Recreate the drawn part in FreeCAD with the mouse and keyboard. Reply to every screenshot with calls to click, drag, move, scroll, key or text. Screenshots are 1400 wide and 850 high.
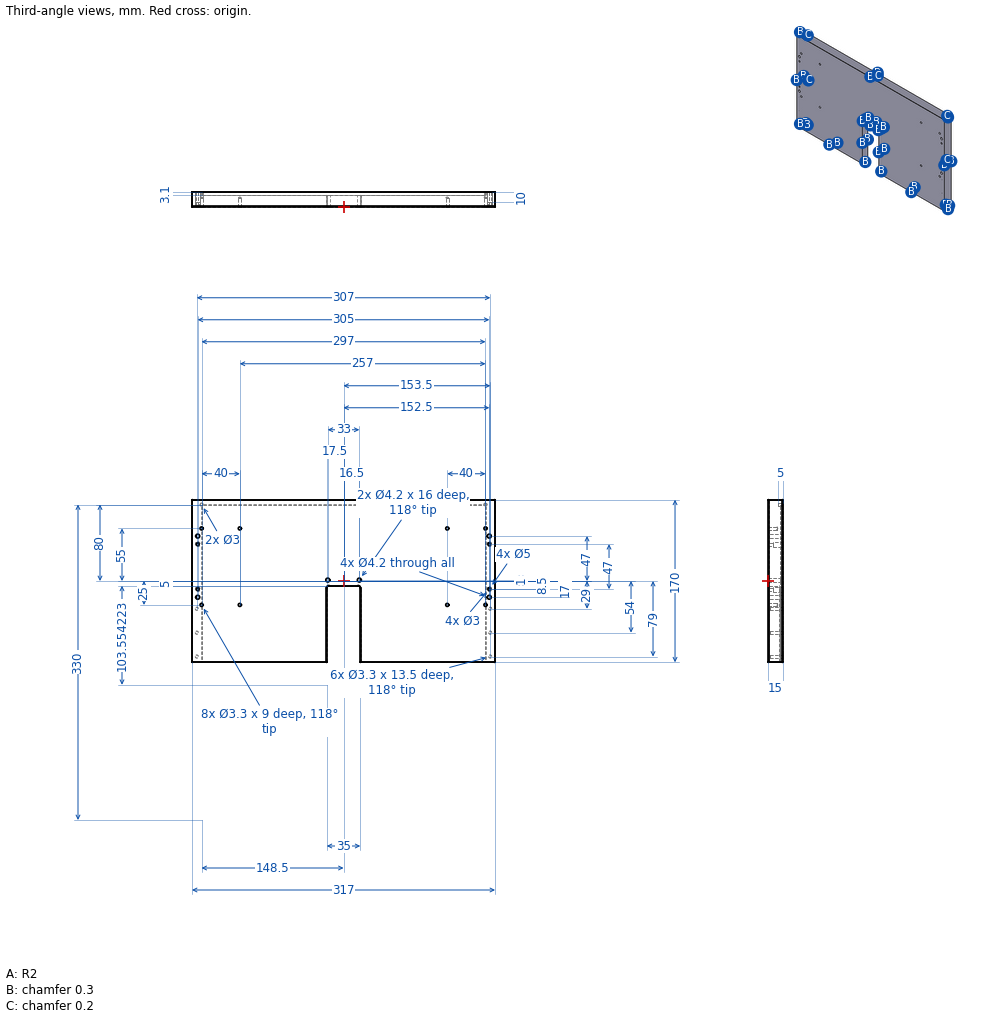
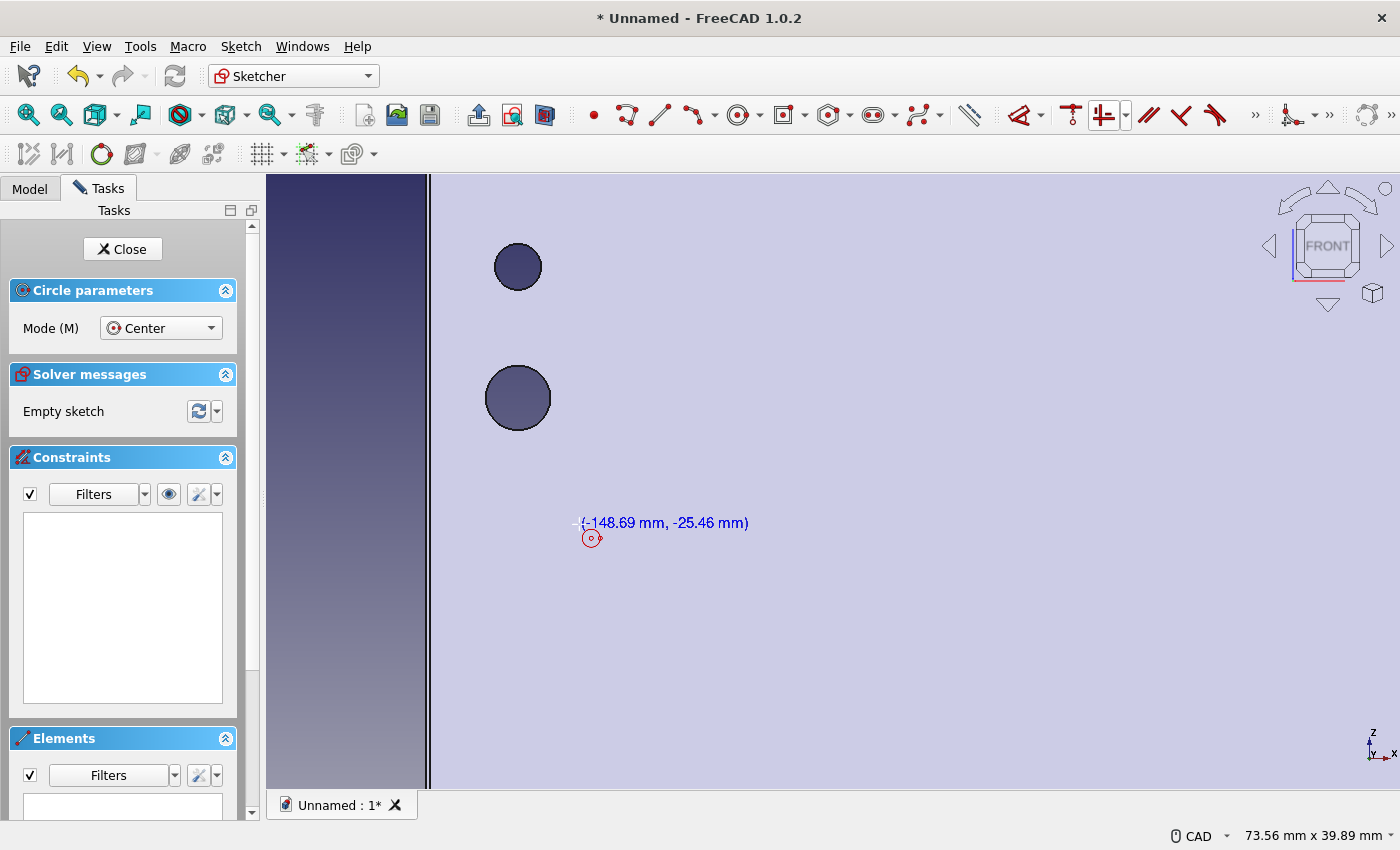
scroll(435, 572, down, 10)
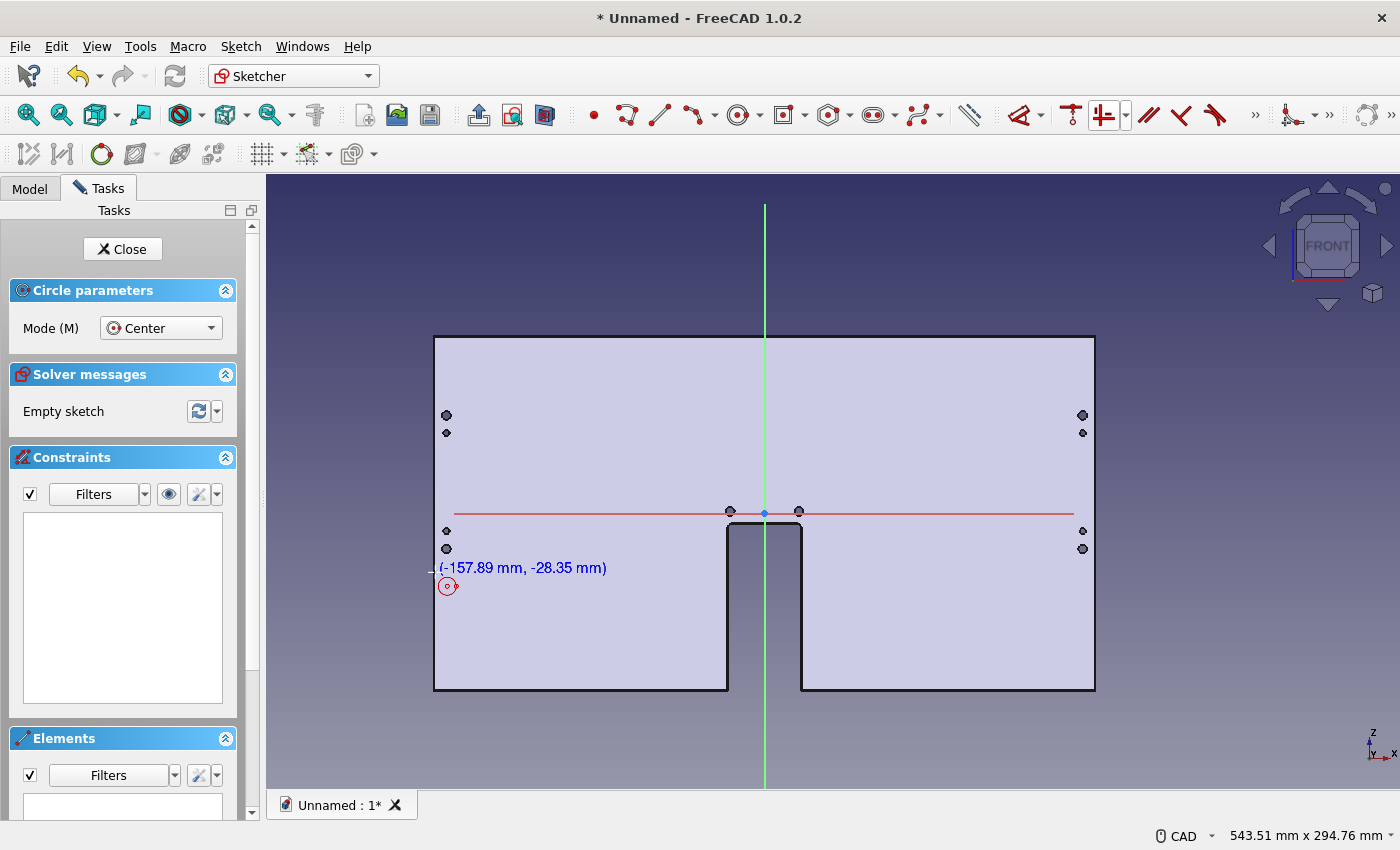
click(455, 566)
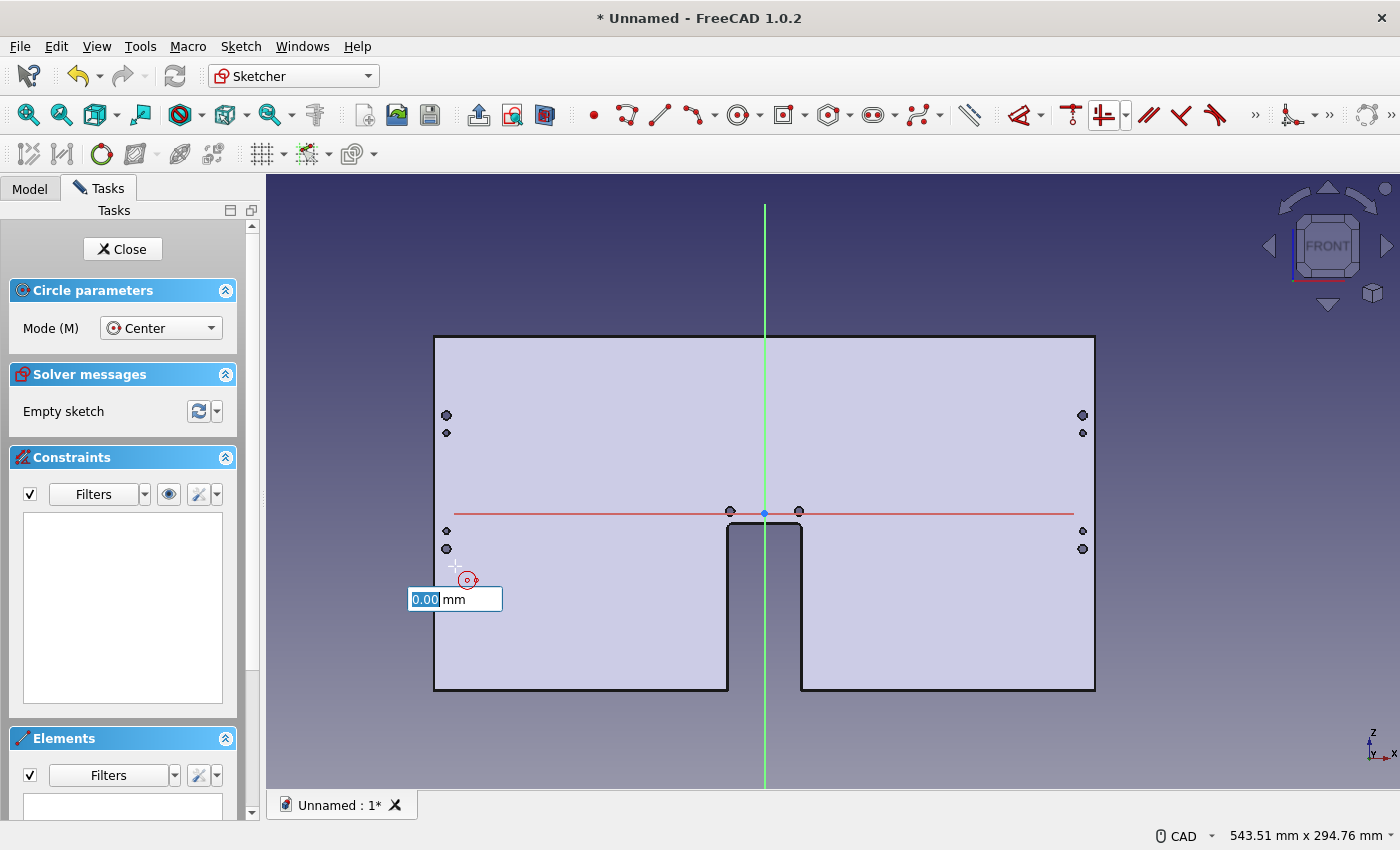
scroll(457, 563, up, 8)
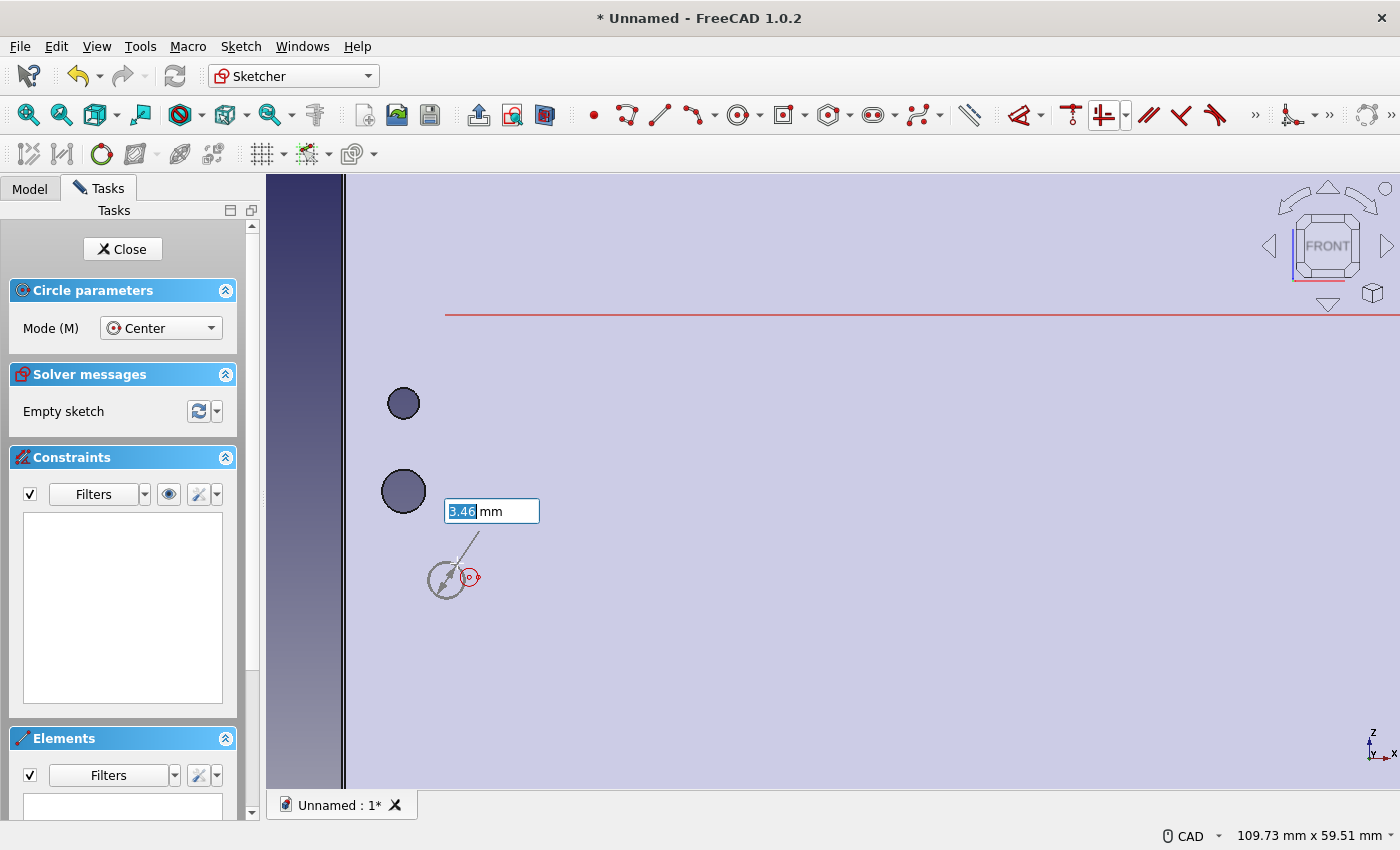
click(457, 562)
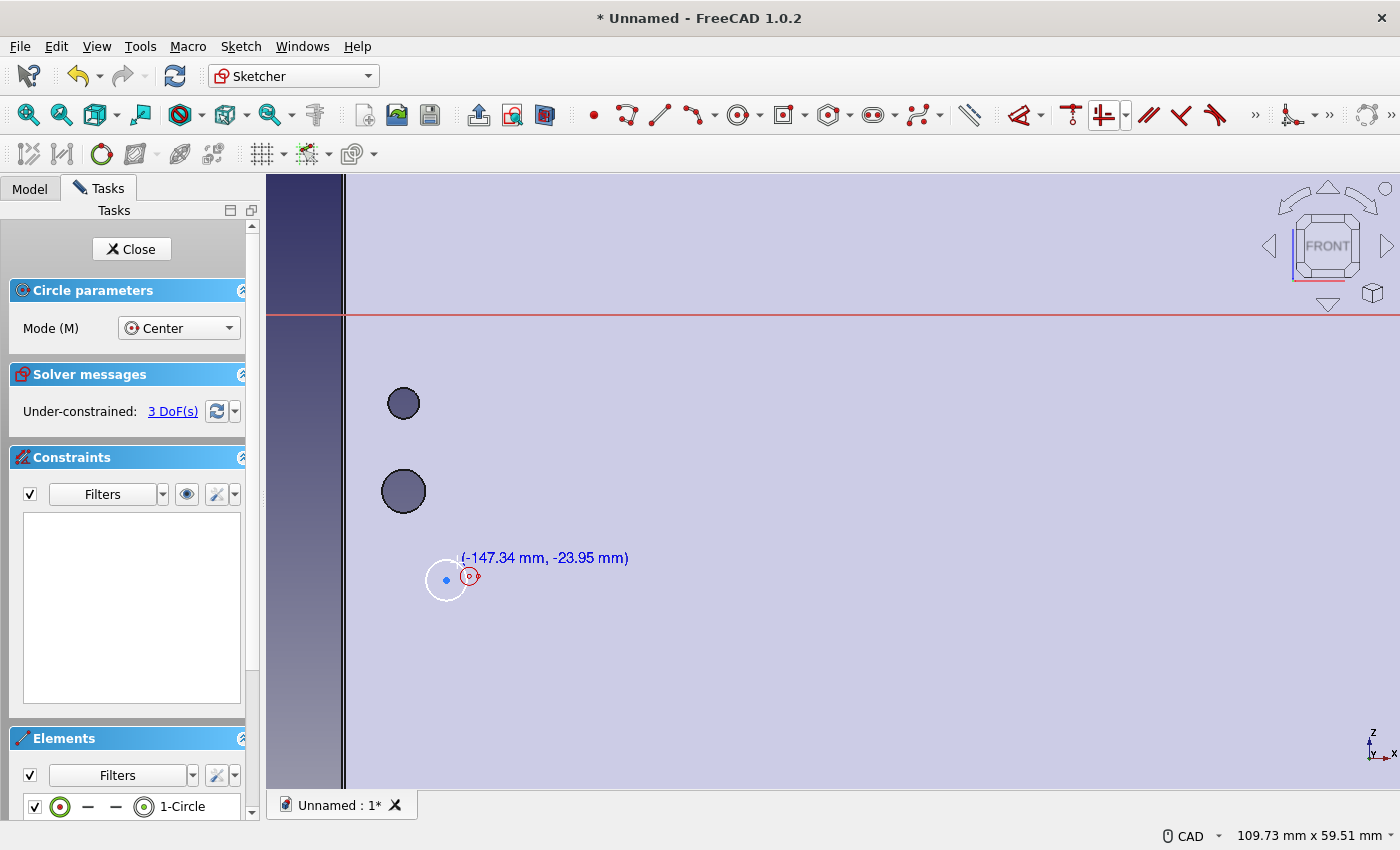
scroll(457, 563, down, 8)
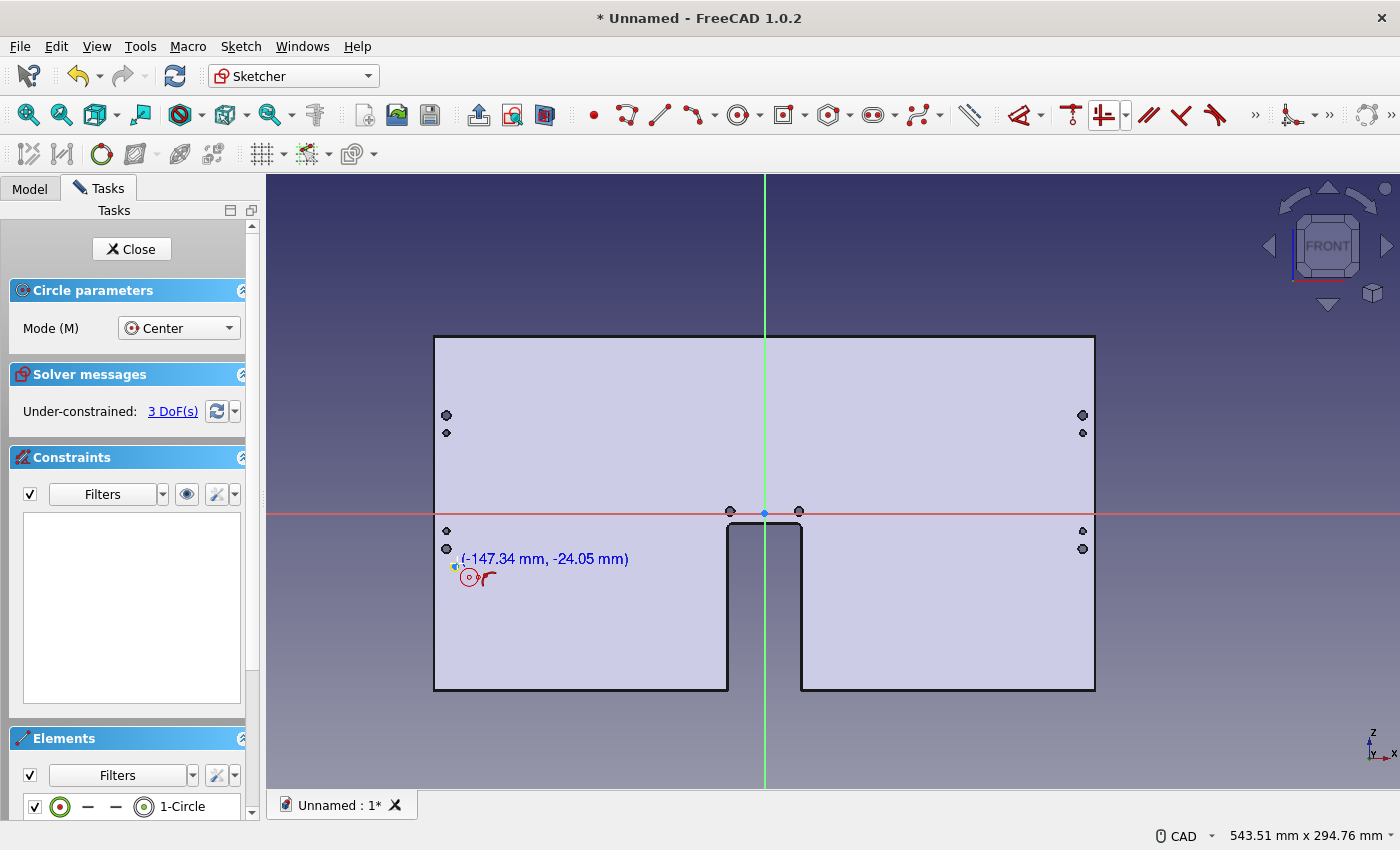
scroll(455, 399, up, 10)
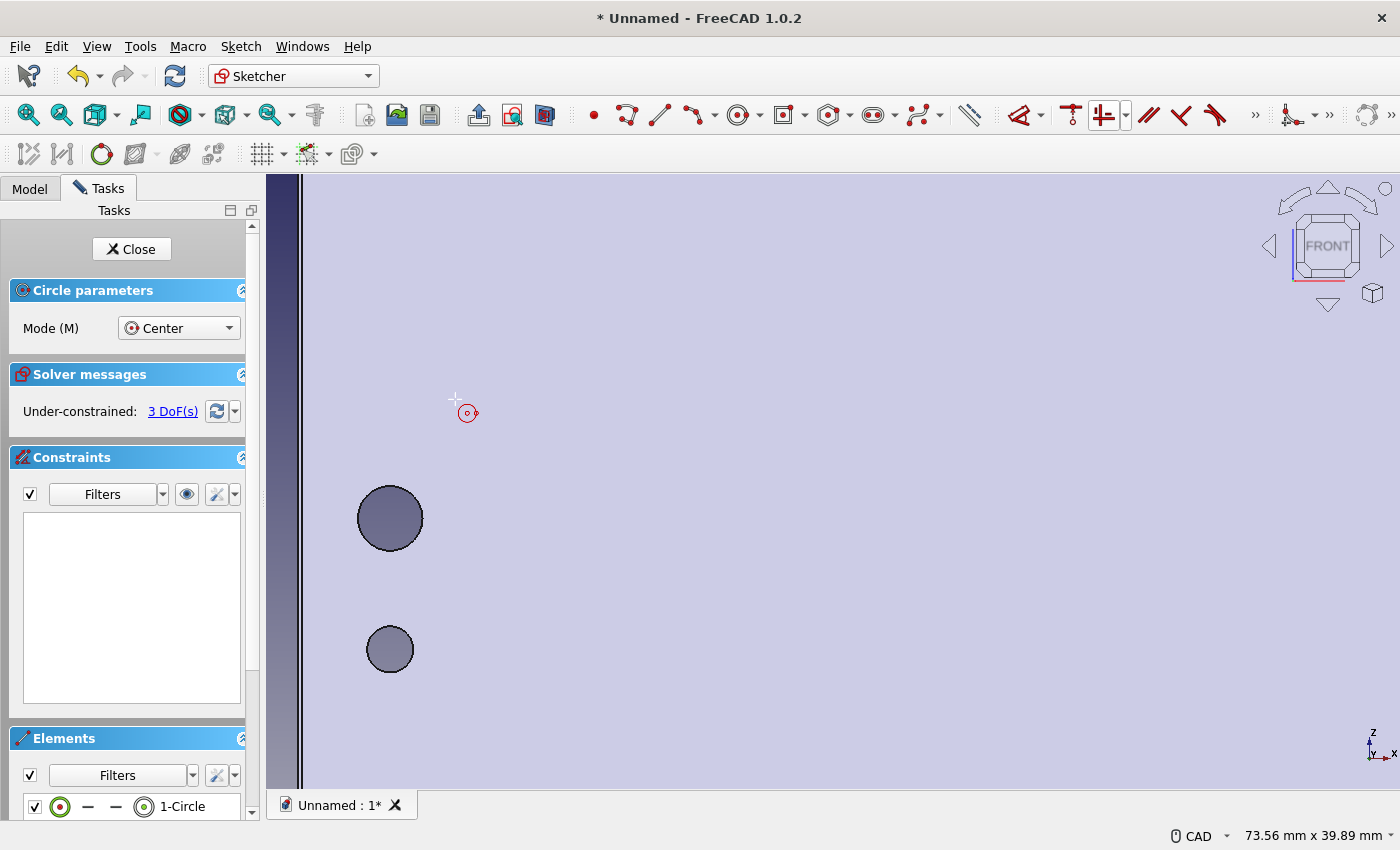
scroll(455, 399, down, 10)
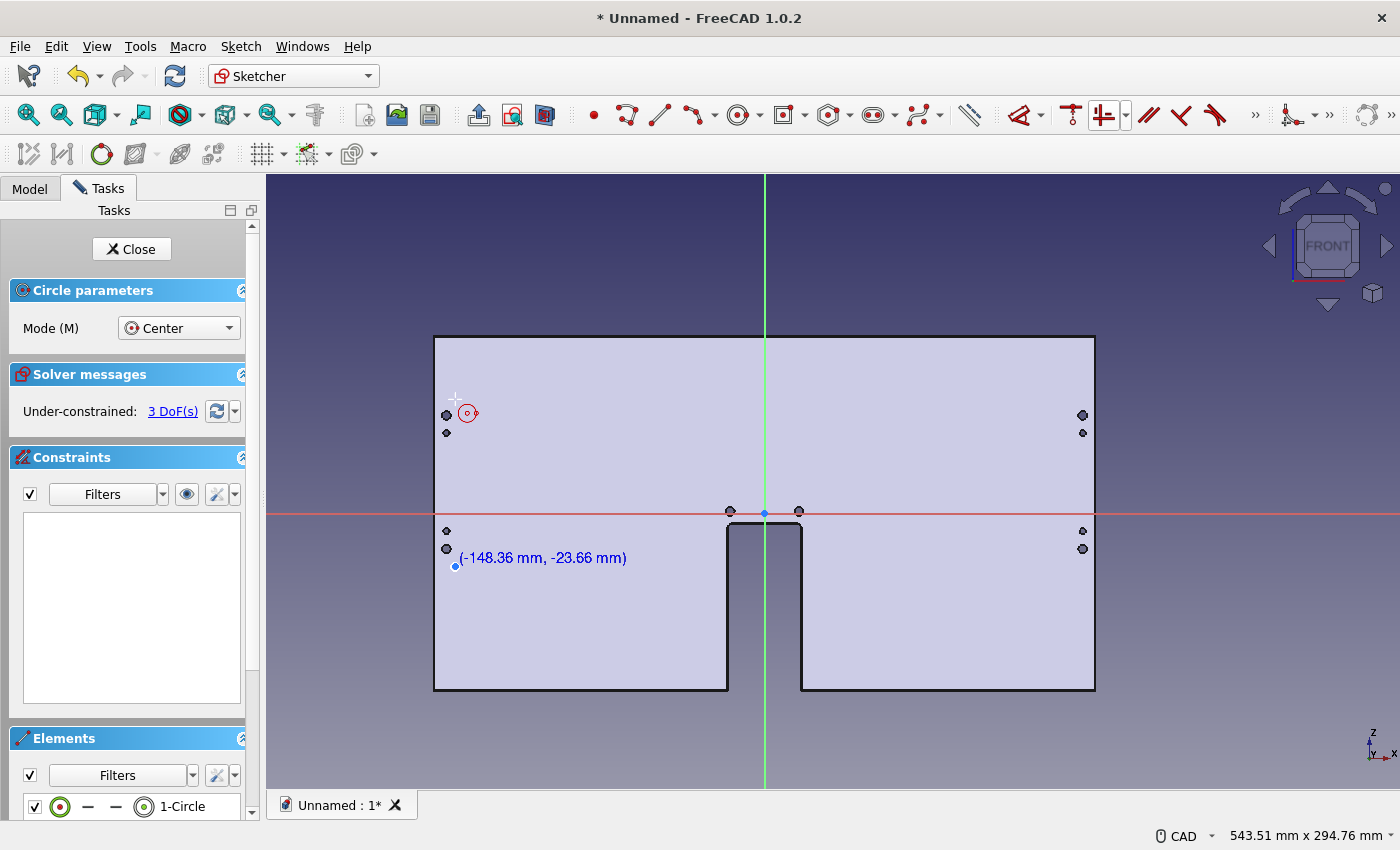
click(455, 399)